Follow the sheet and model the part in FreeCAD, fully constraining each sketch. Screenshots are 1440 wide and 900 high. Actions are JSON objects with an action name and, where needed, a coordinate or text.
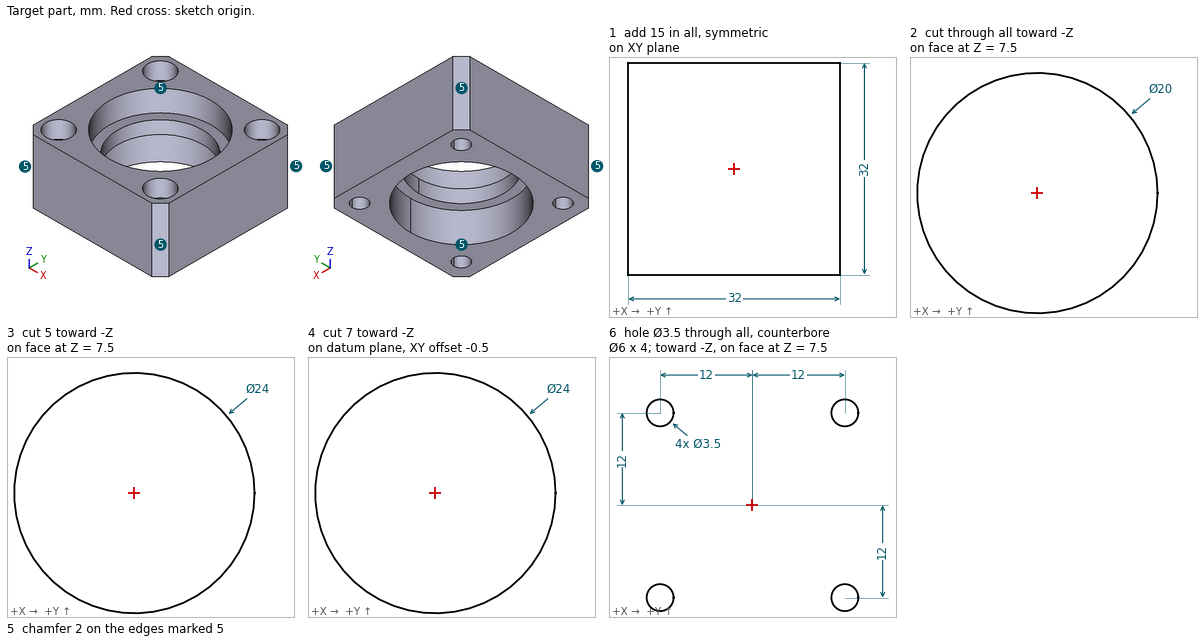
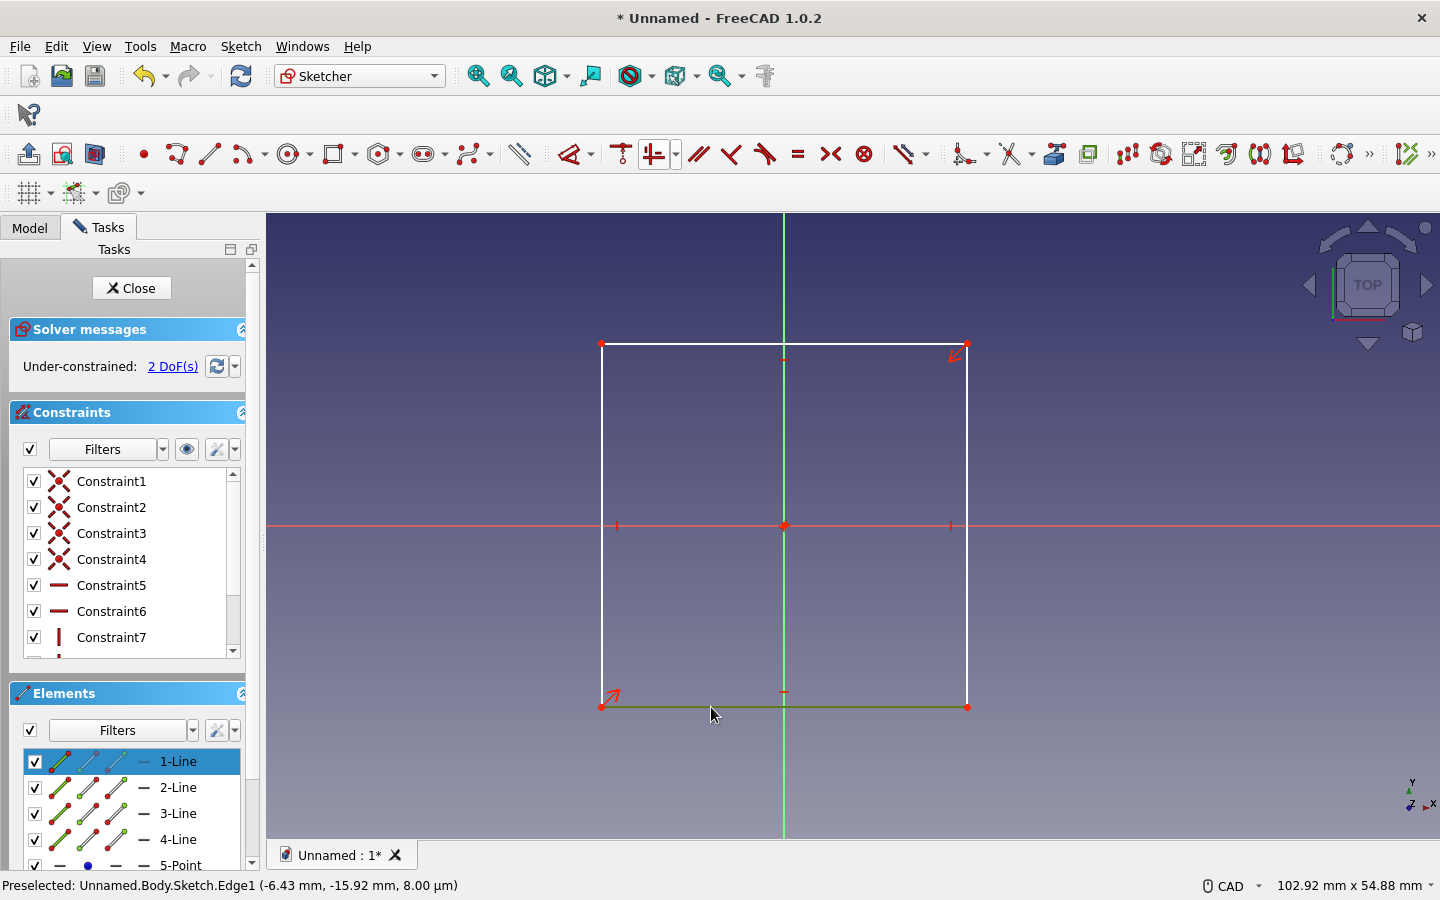
{"action": "key", "text": "l"}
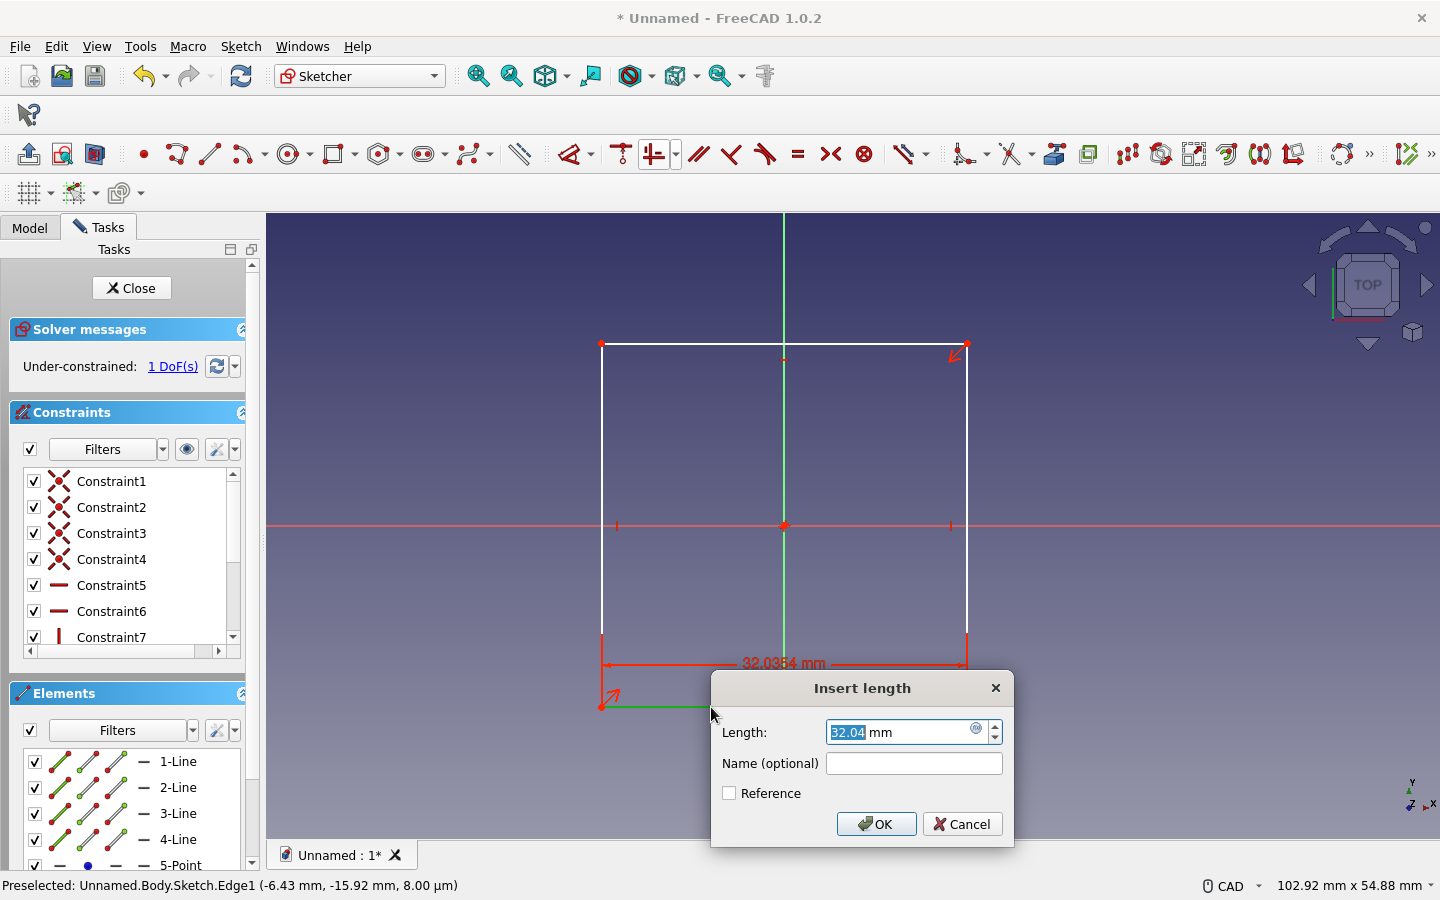
{"action": "type", "text": "32"}
{"action": "key", "text": "Return"}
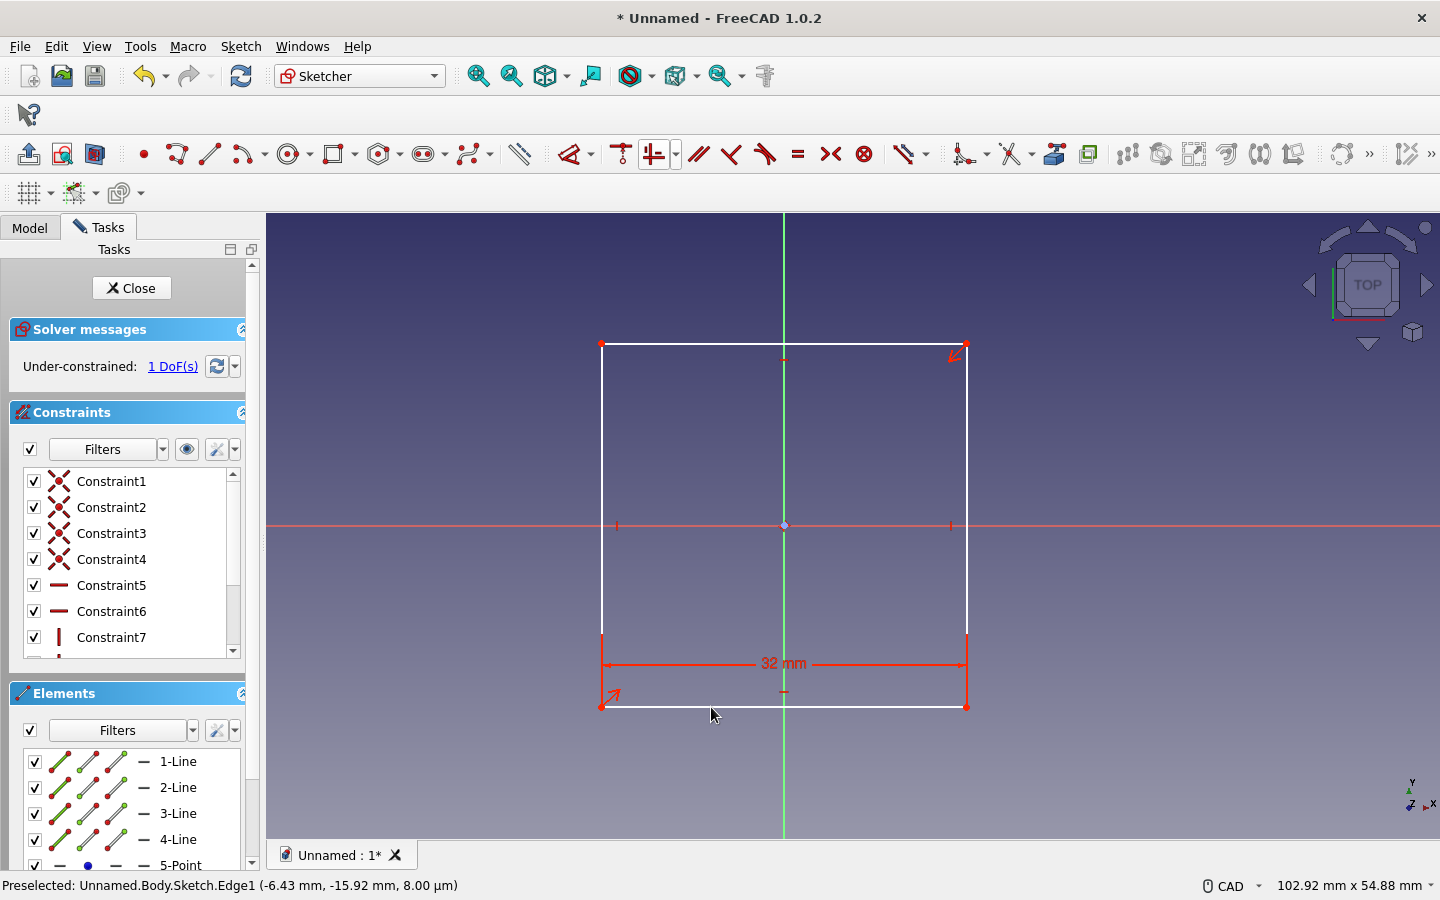
{"action": "left_click", "coordinate": [967, 598]}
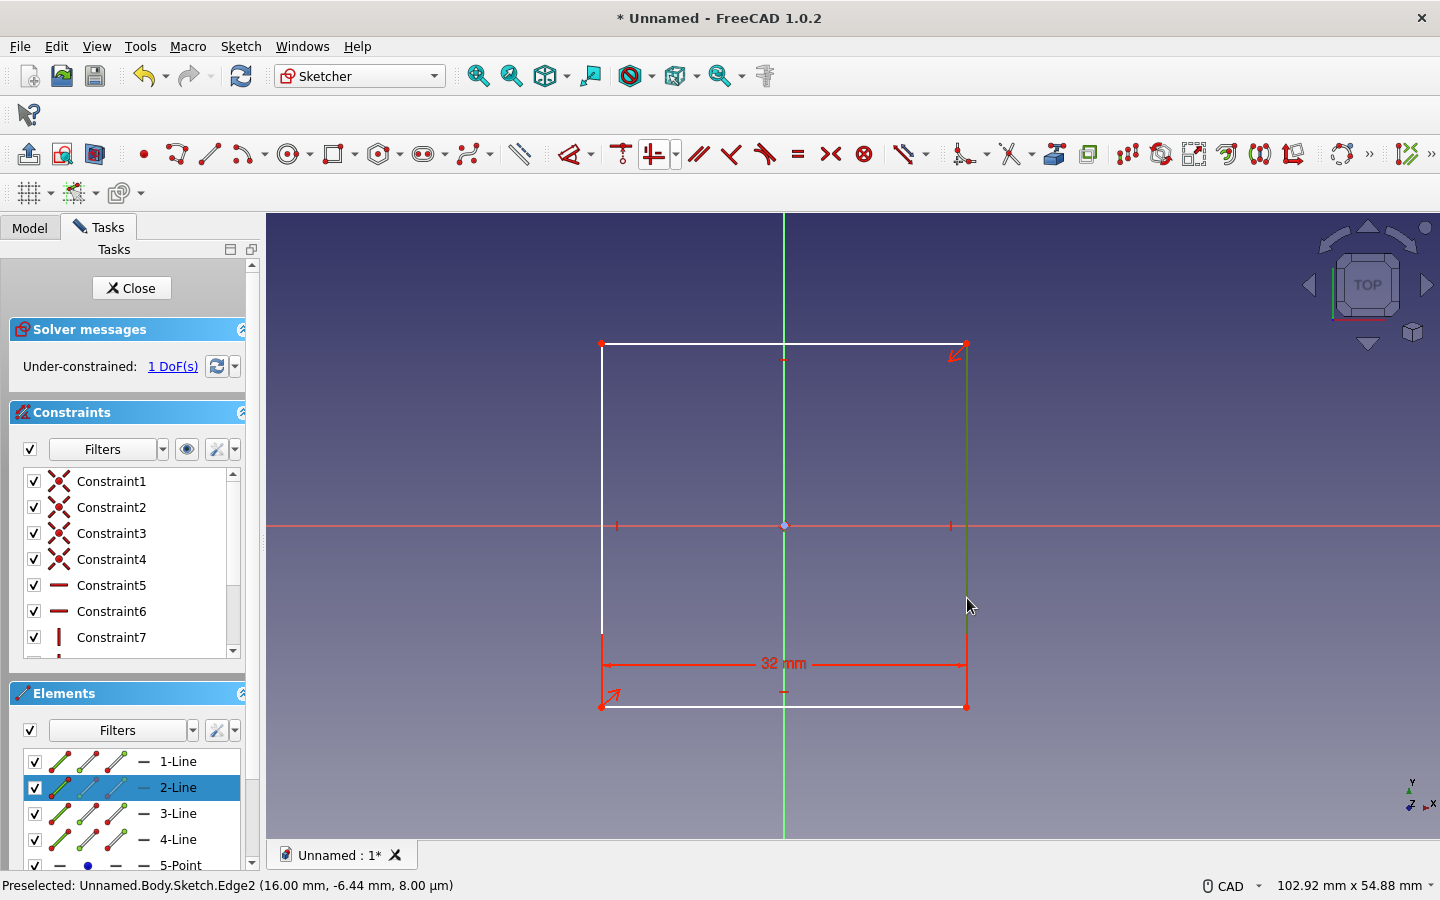
{"action": "left_click", "coordinate": [590, 154]}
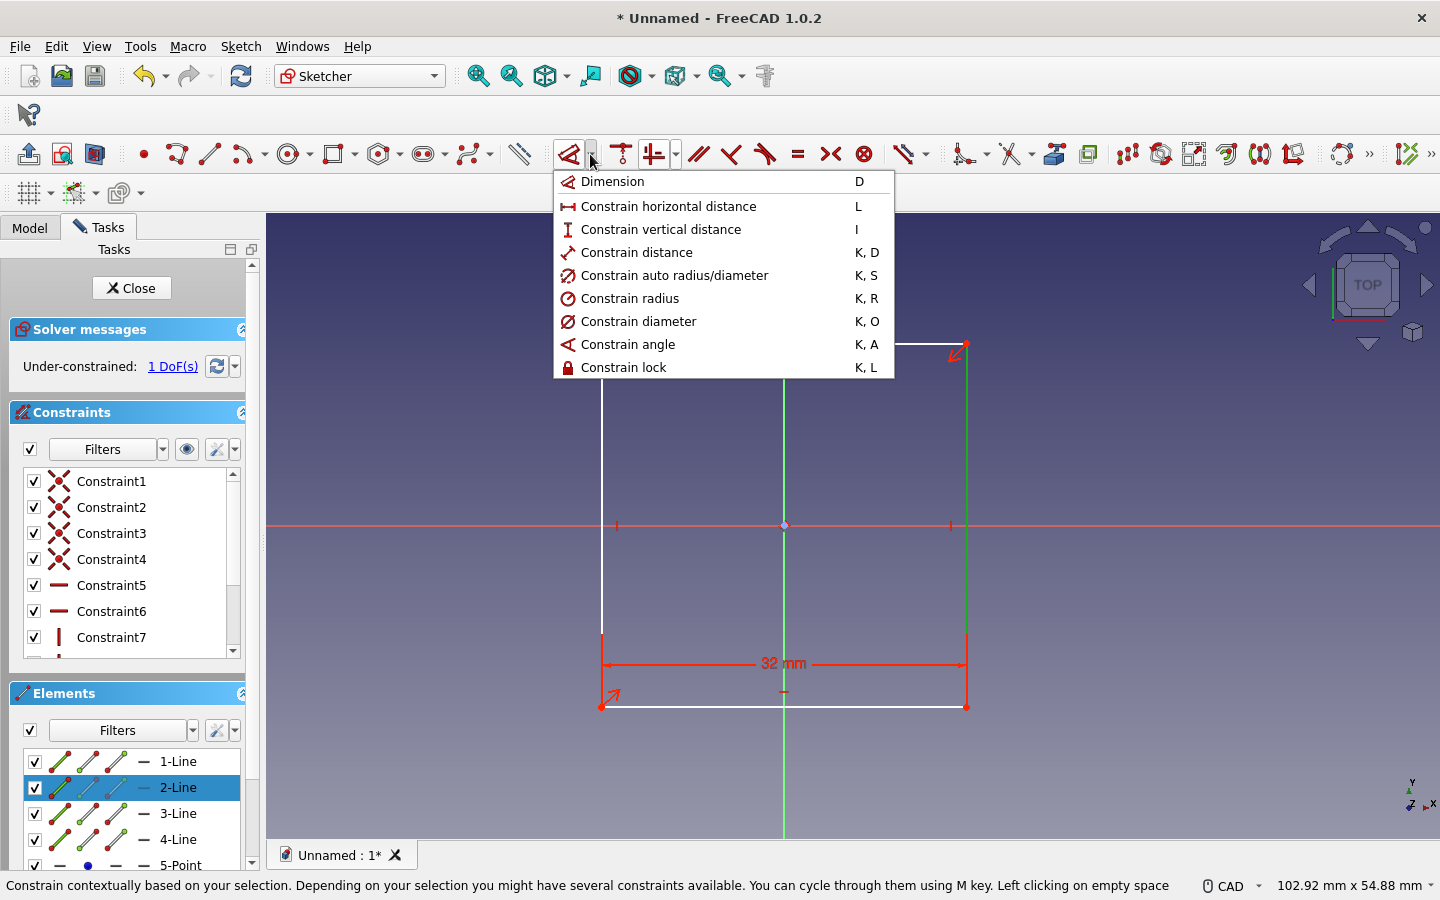
{"action": "left_click", "coordinate": [724, 230]}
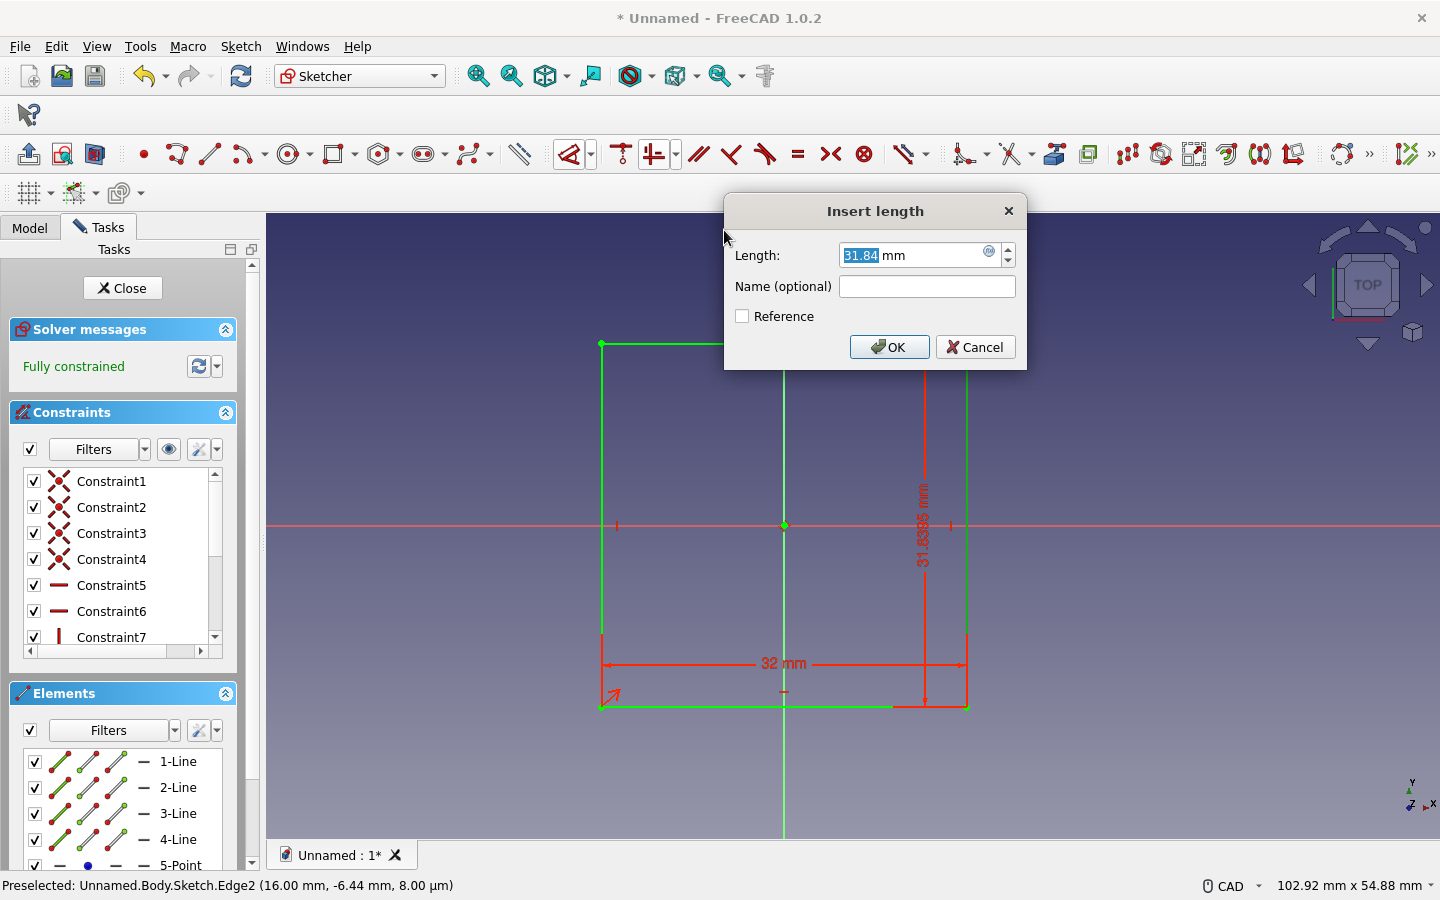
{"action": "type", "text": "32"}
{"action": "key", "text": "Return"}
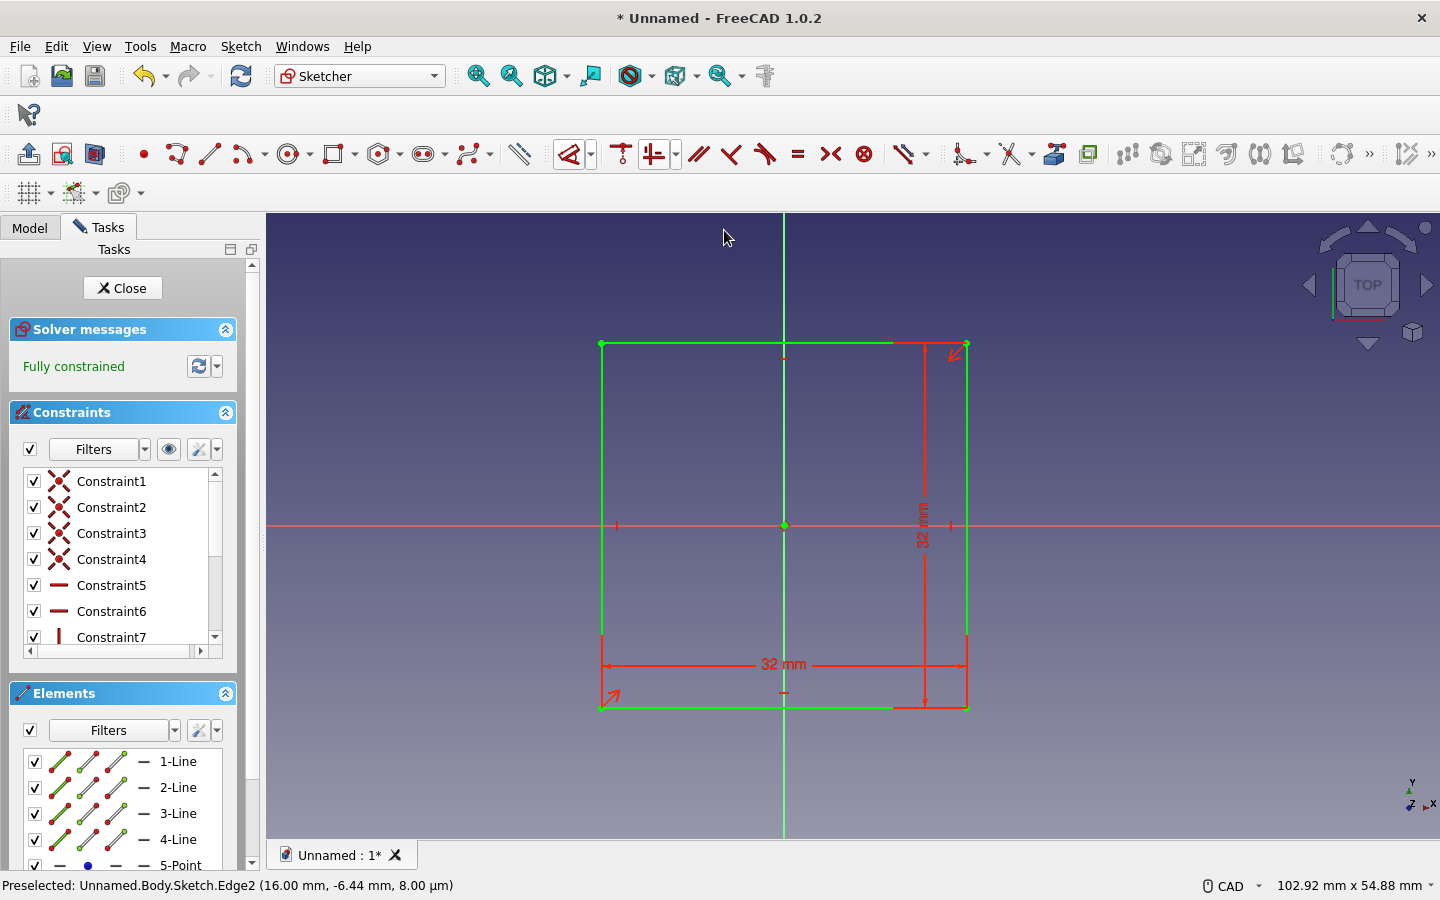
{"action": "left_click", "coordinate": [123, 288]}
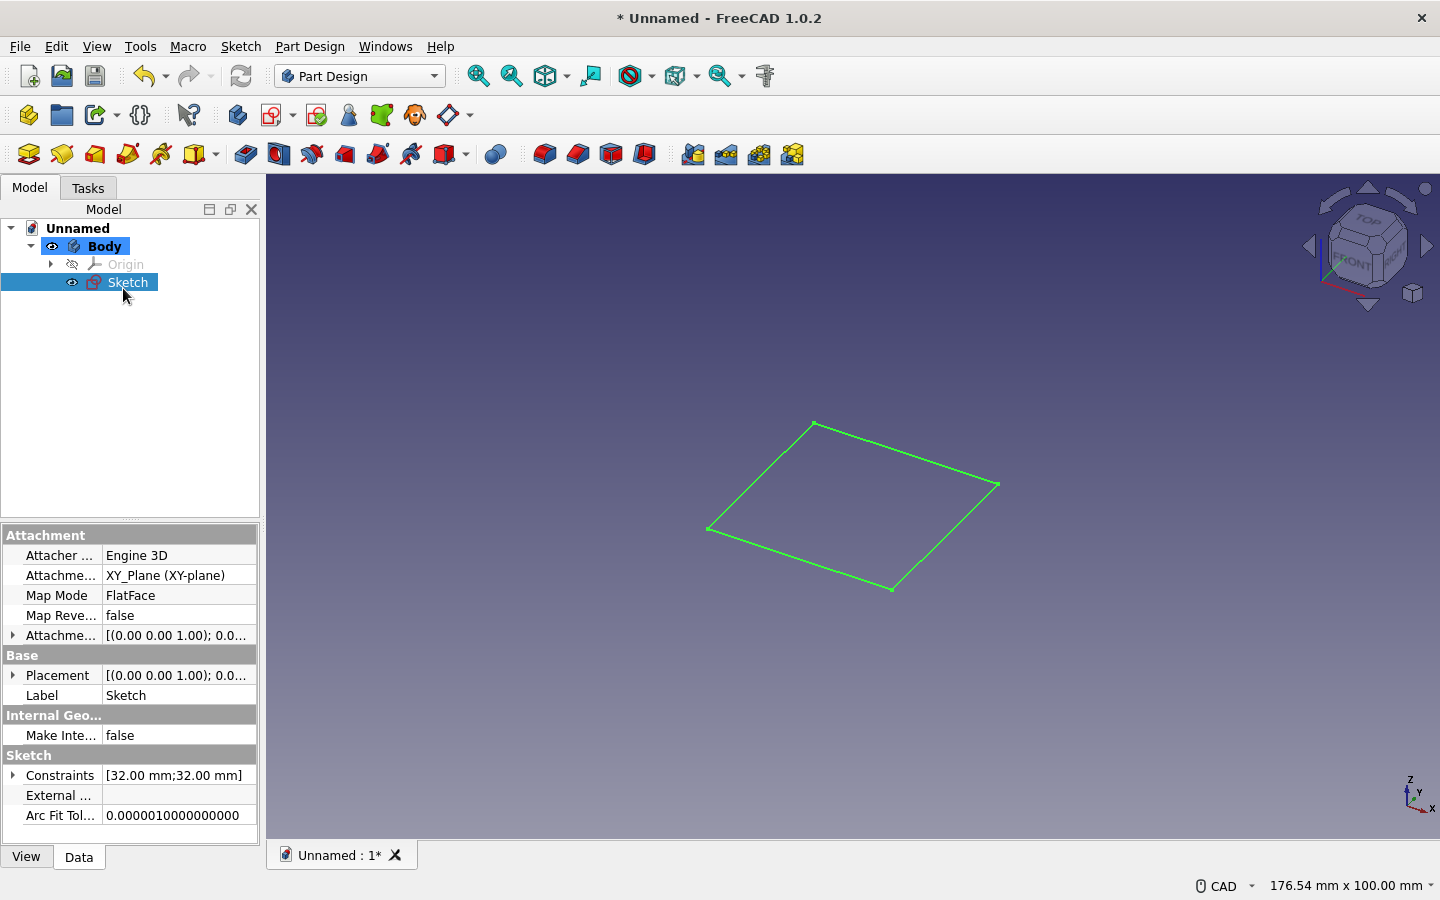
{"action": "left_click", "coordinate": [29, 154]}